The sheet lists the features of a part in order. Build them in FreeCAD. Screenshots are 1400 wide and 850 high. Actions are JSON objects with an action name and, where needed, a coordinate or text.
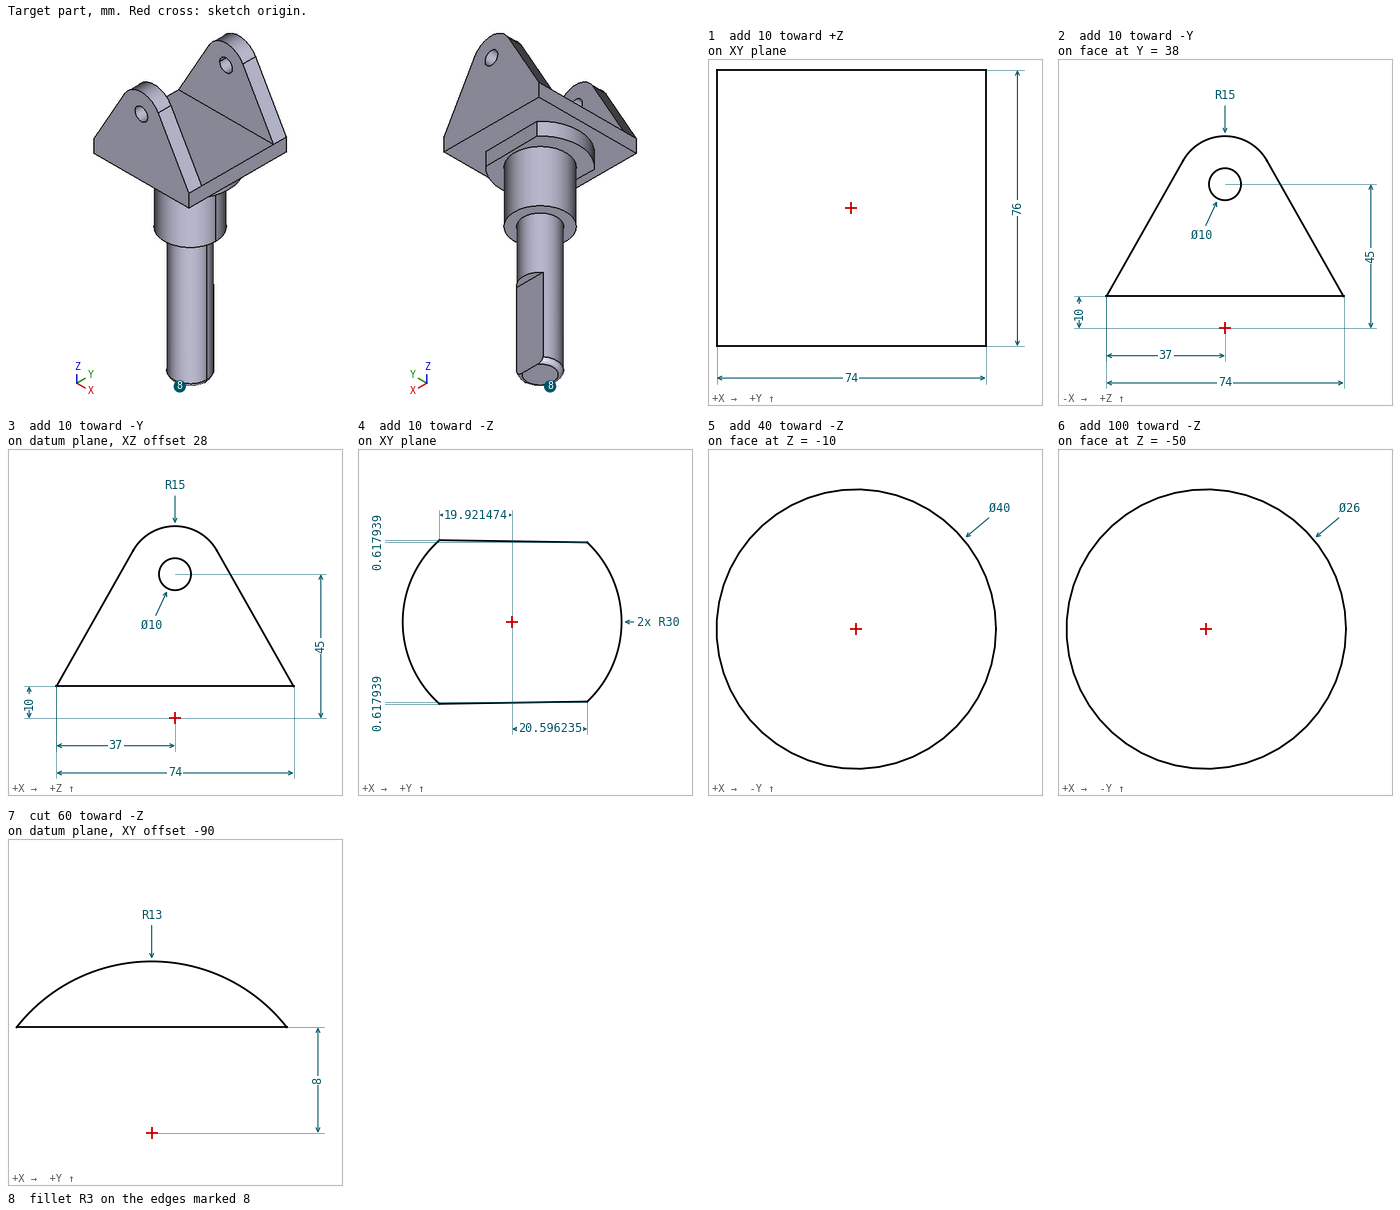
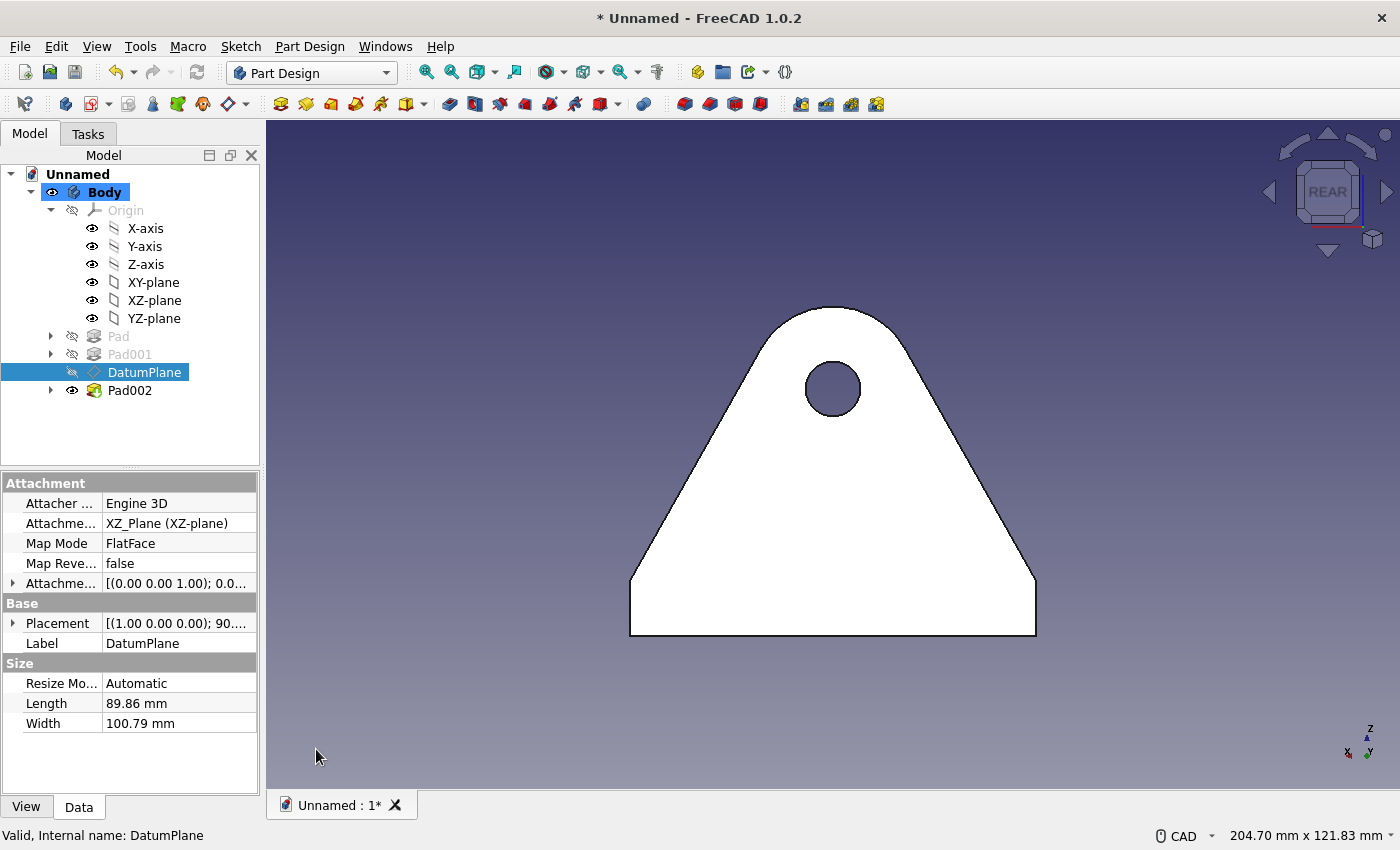
{"action": "left_click", "coordinate": [90, 104]}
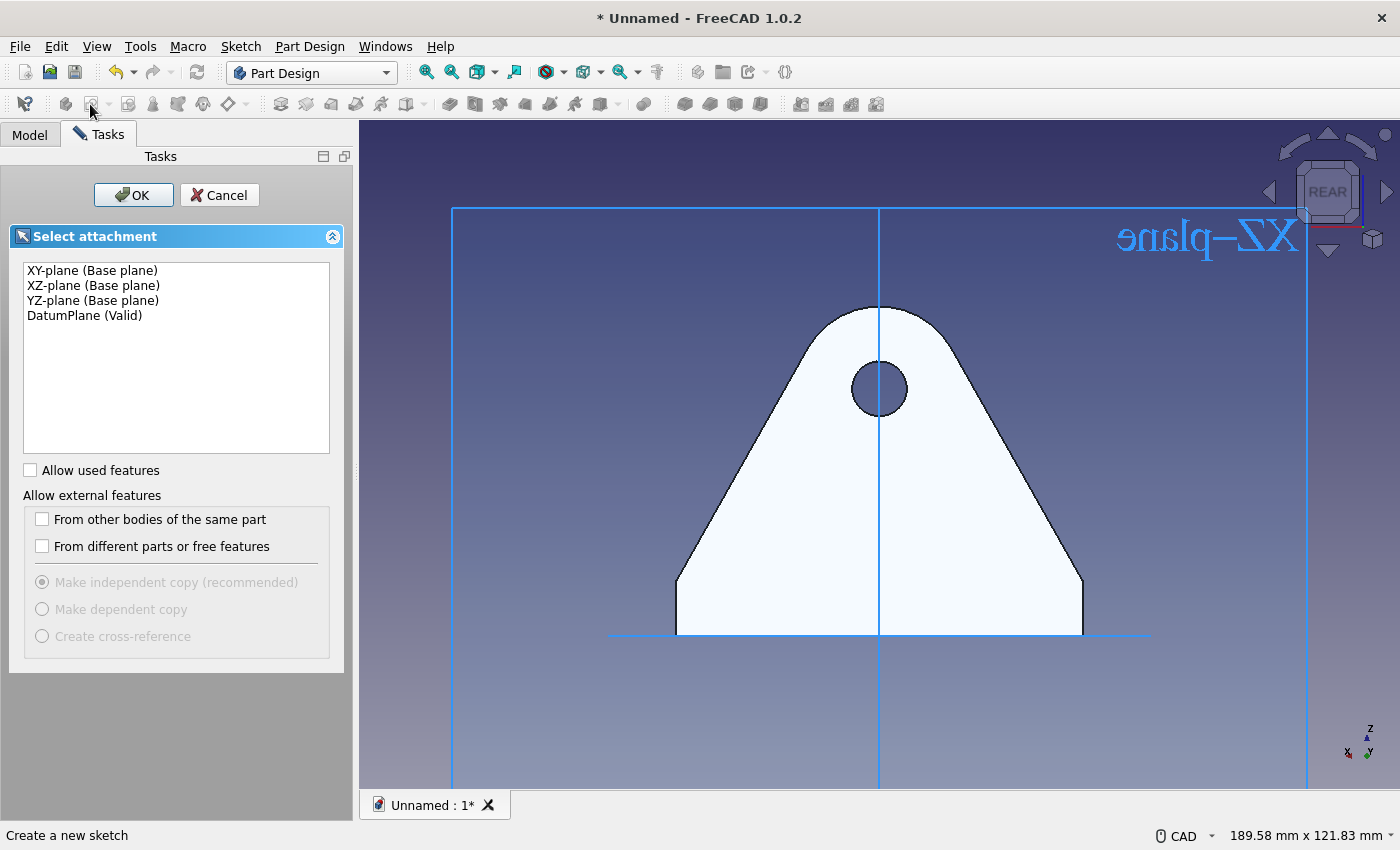
{"action": "left_click", "coordinate": [84, 270]}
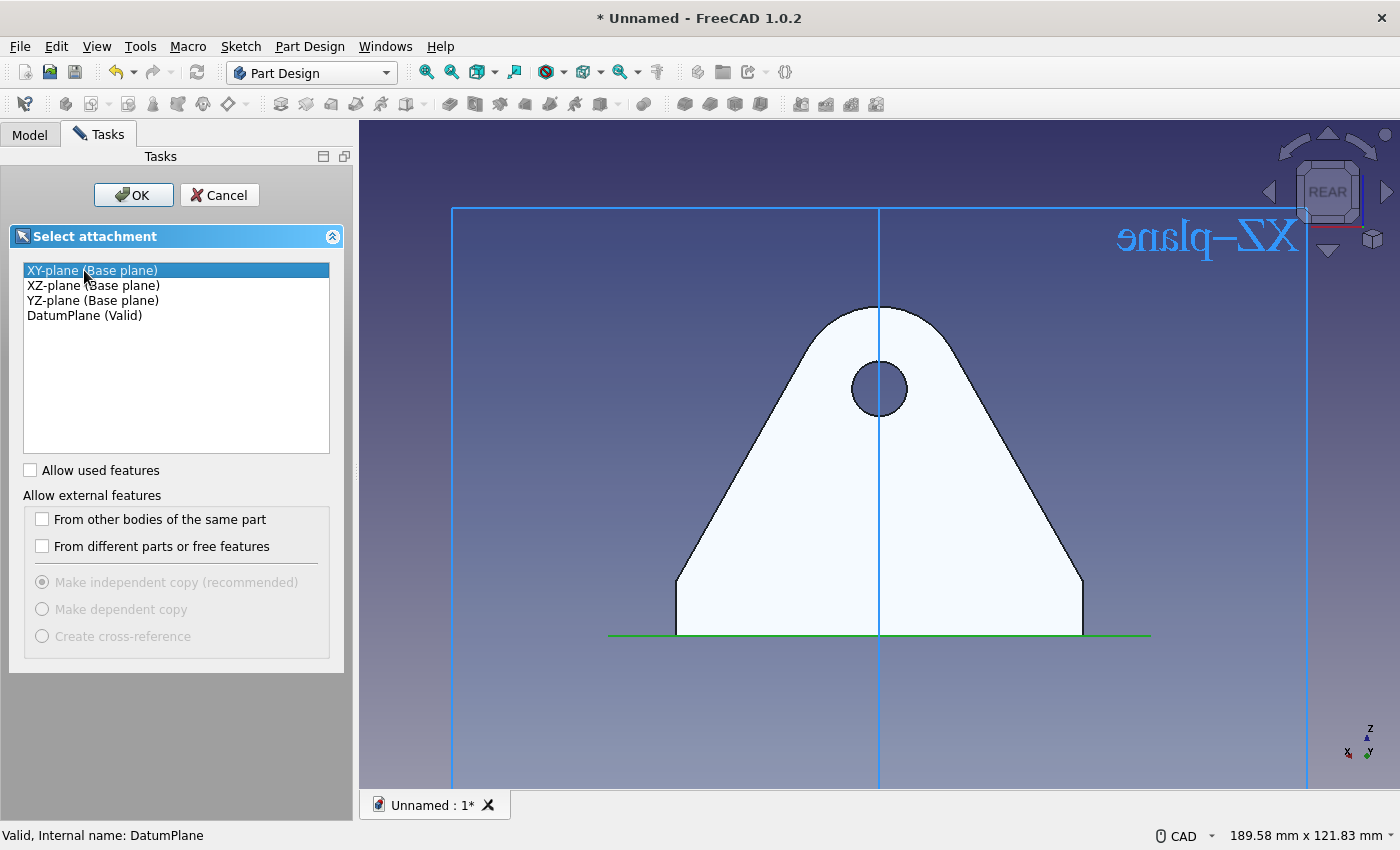
{"action": "left_click", "coordinate": [134, 195]}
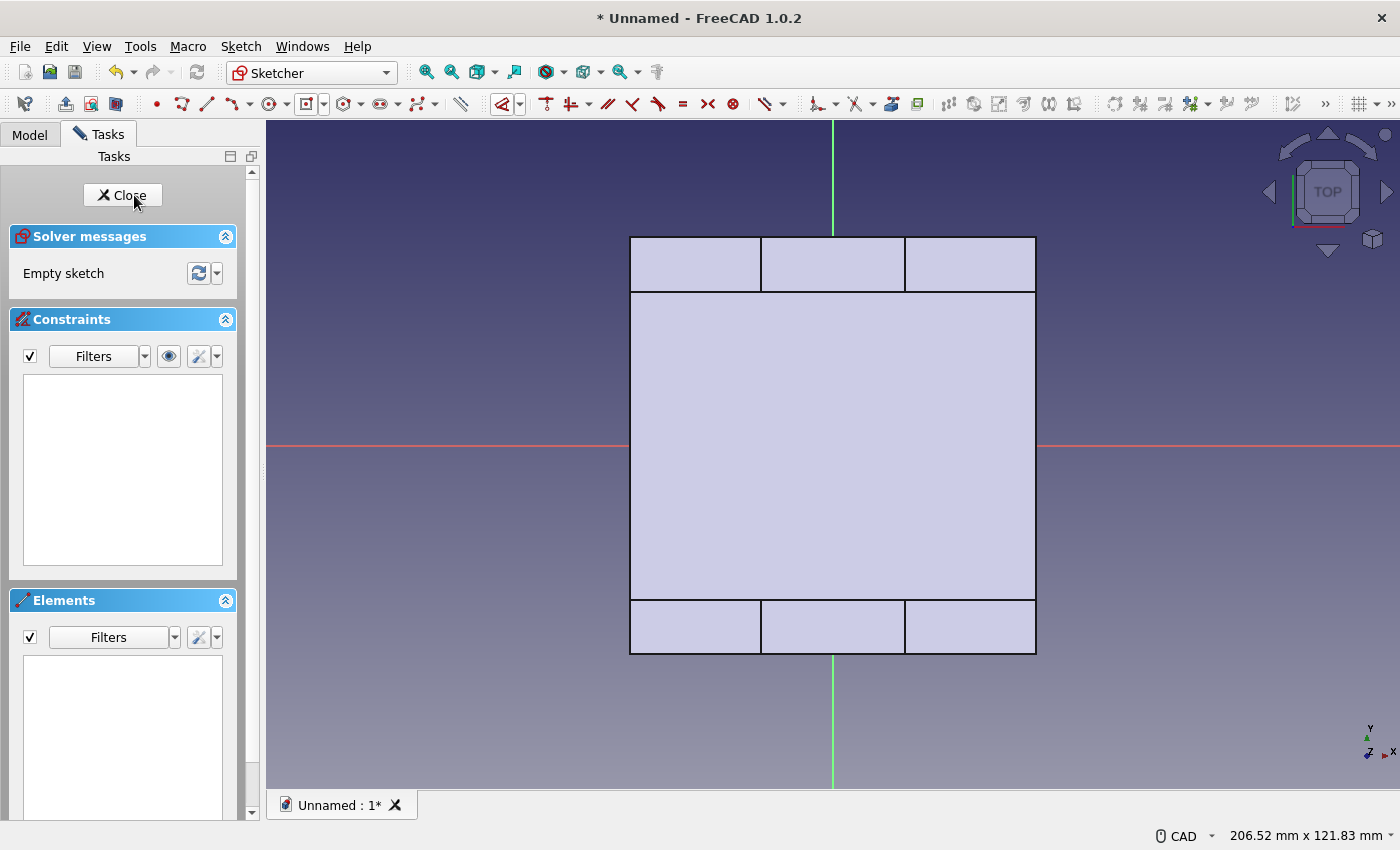
{"action": "left_click", "coordinate": [116, 104]}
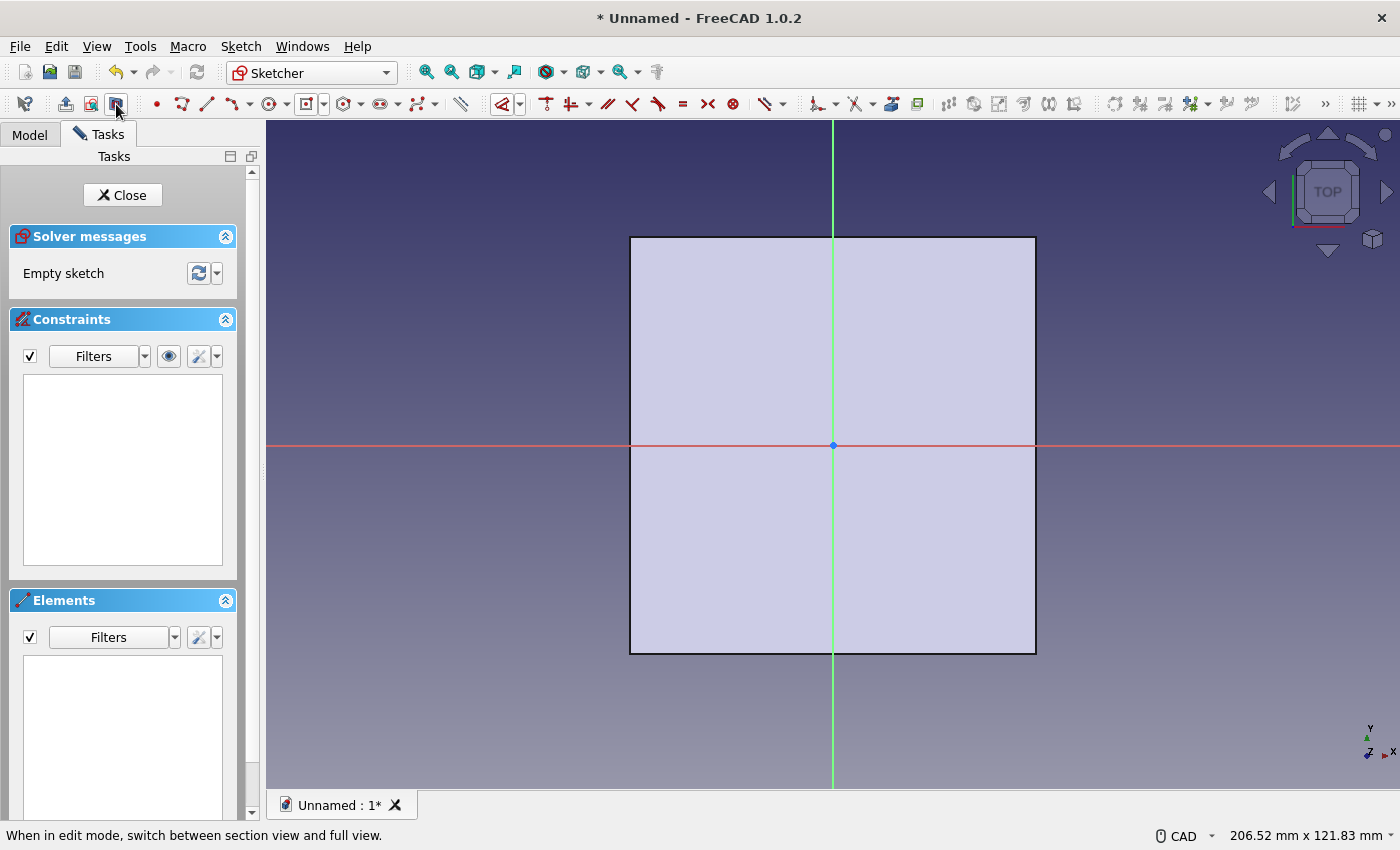
{"action": "scroll", "coordinate": [916, 435], "scroll_direction": "up", "scroll_amount": 3}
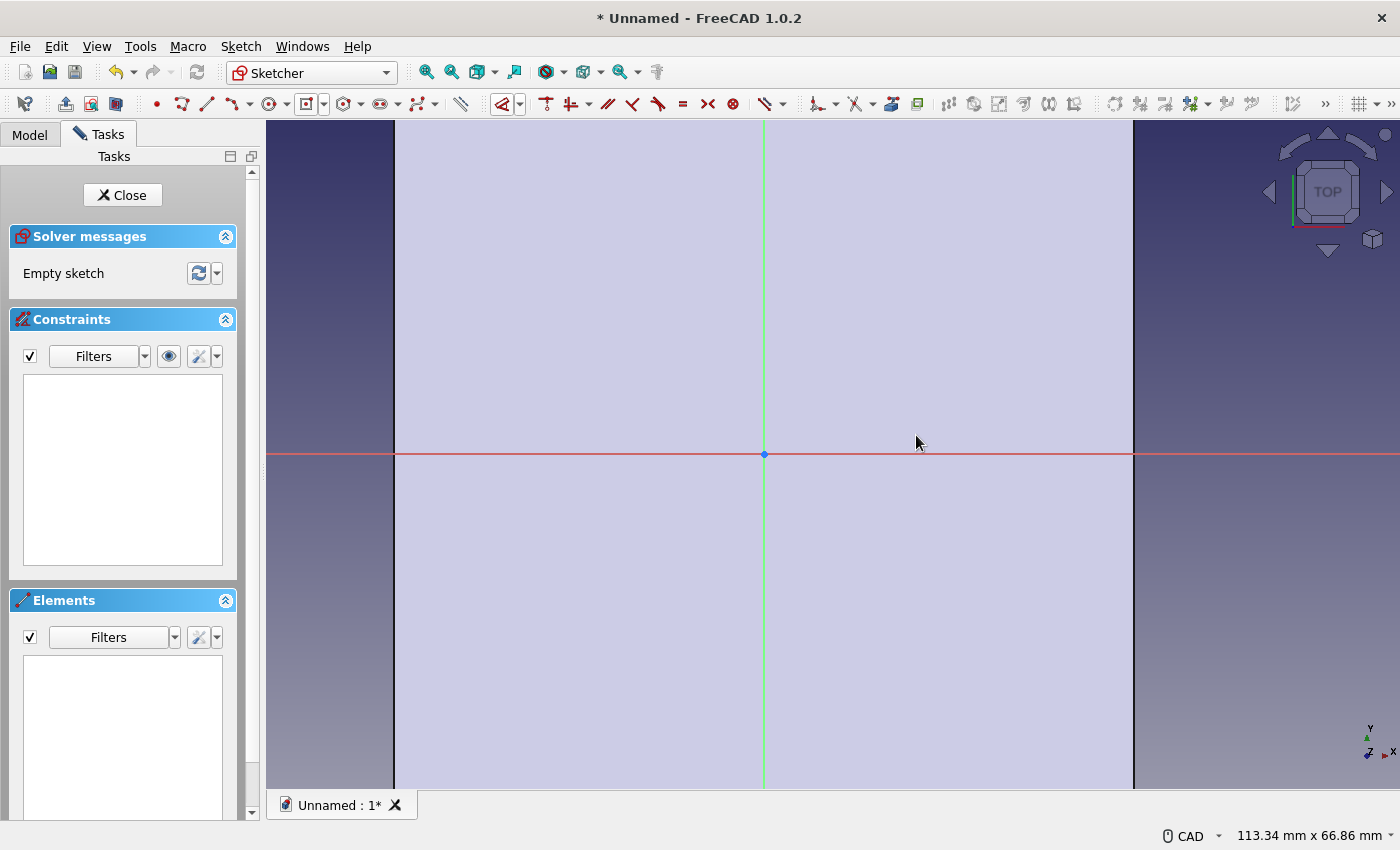
{"action": "left_click", "coordinate": [207, 104]}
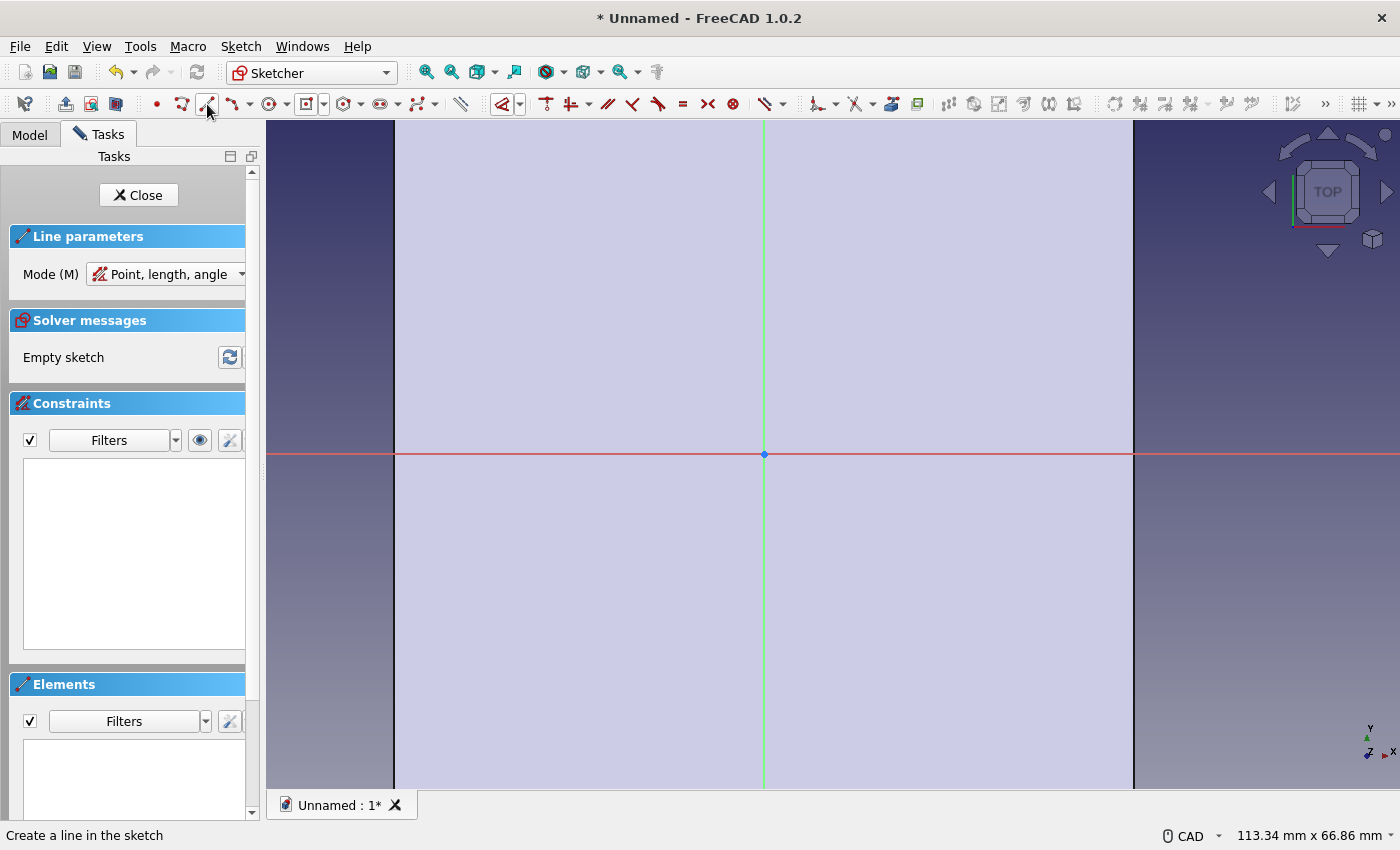
{"action": "left_click", "coordinate": [565, 230]}
{"action": "left_click", "coordinate": [970, 250]}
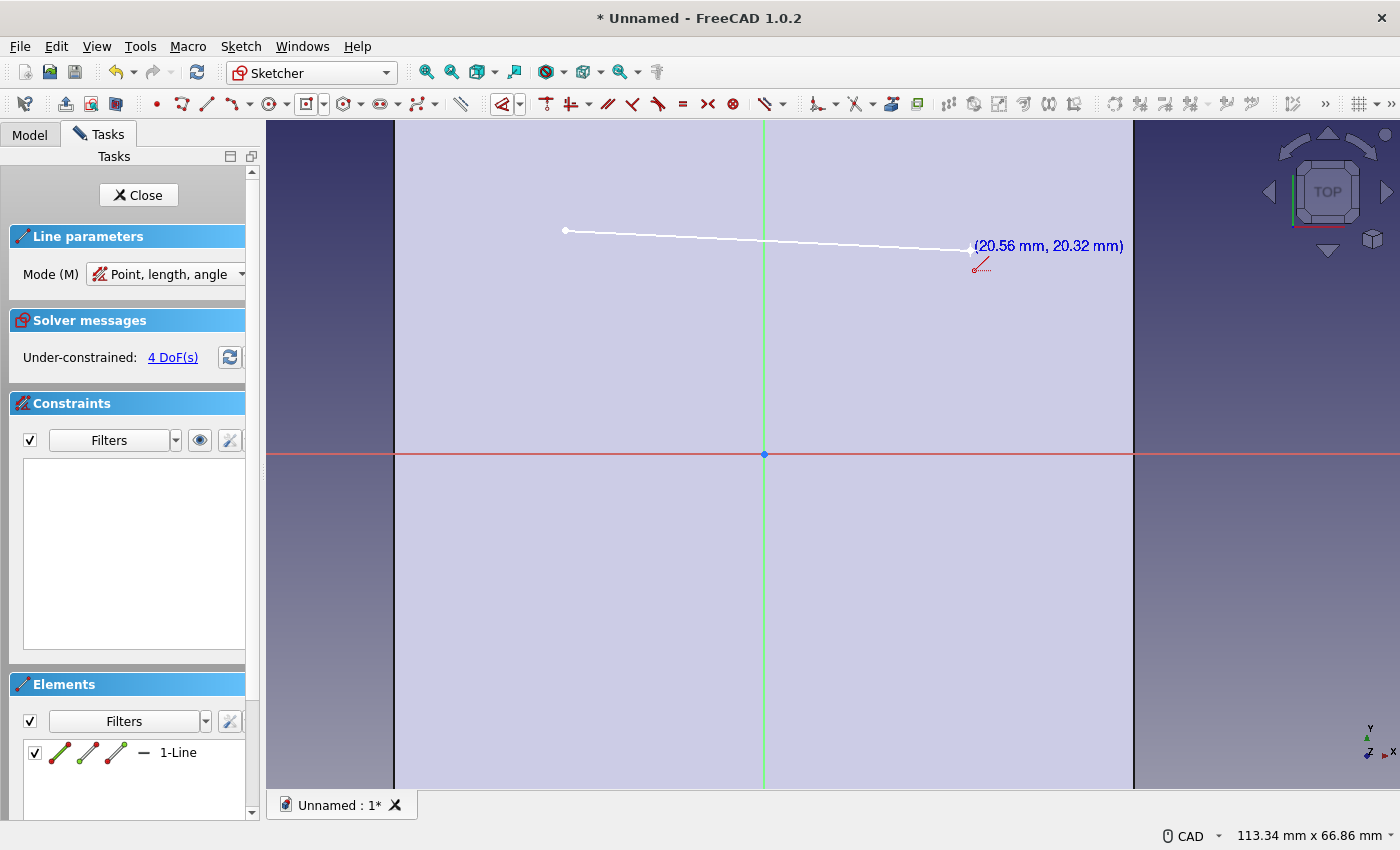
{"action": "left_click", "coordinate": [970, 673]}
{"action": "left_click", "coordinate": [565, 693]}